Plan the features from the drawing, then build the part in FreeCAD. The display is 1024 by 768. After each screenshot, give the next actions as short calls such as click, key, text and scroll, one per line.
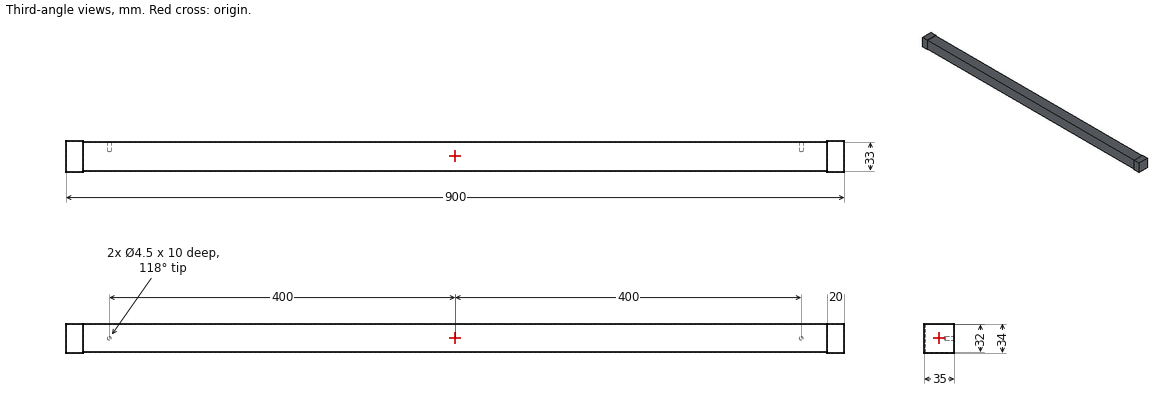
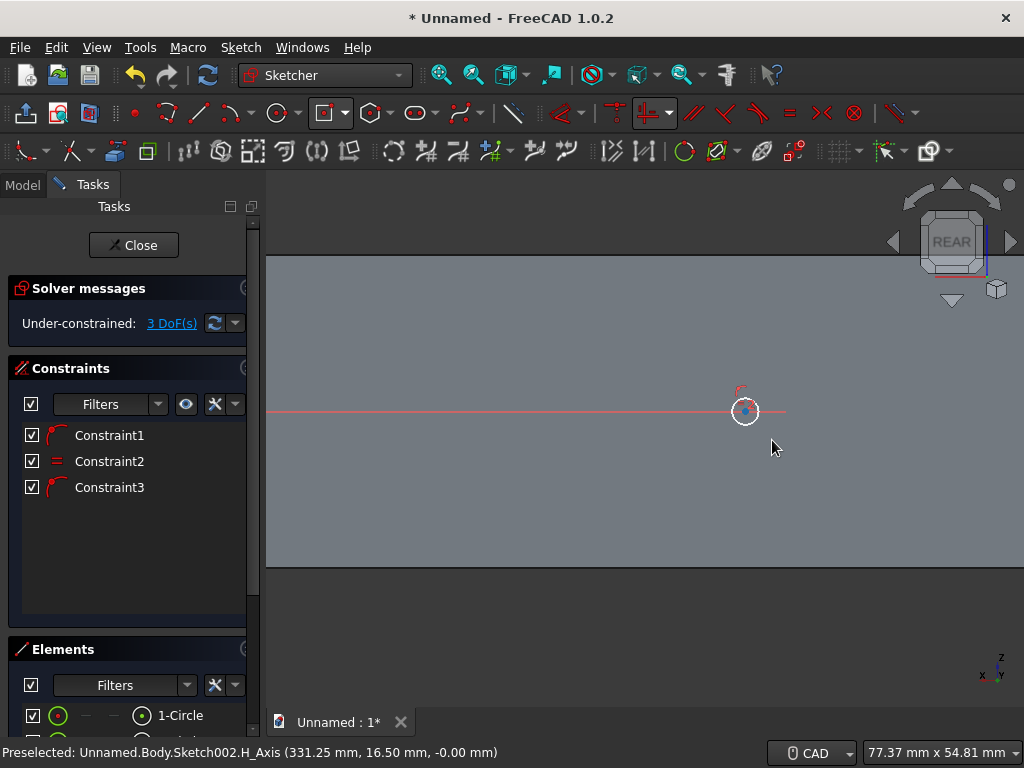
click(755, 421)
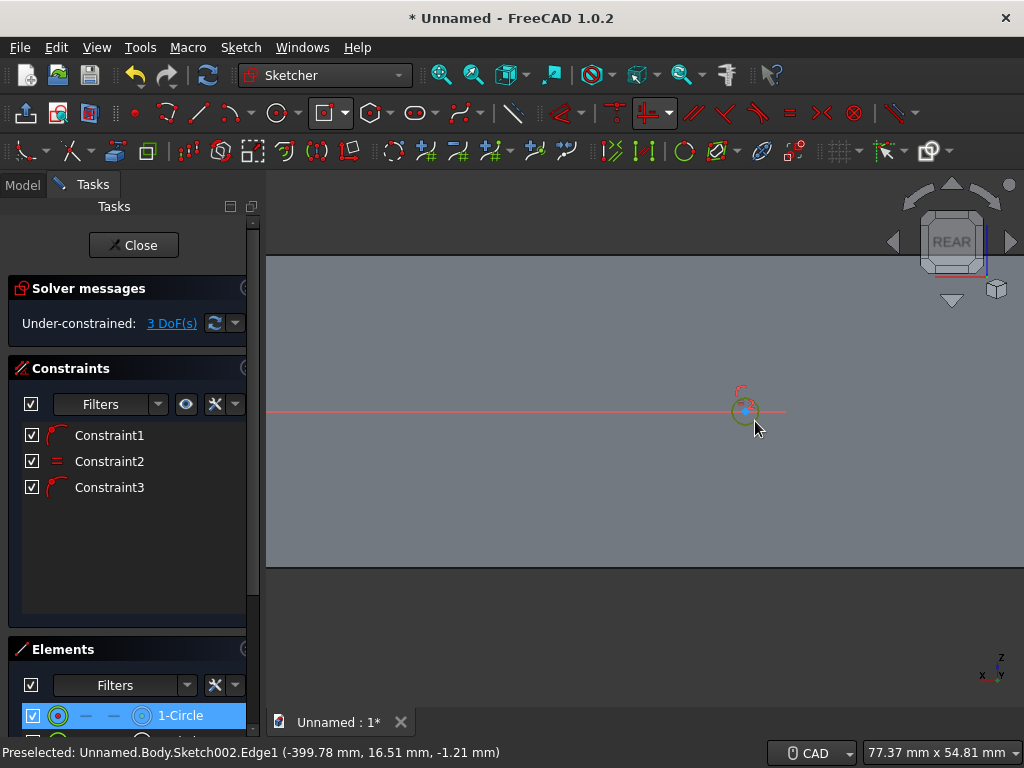
key(k)
key(o)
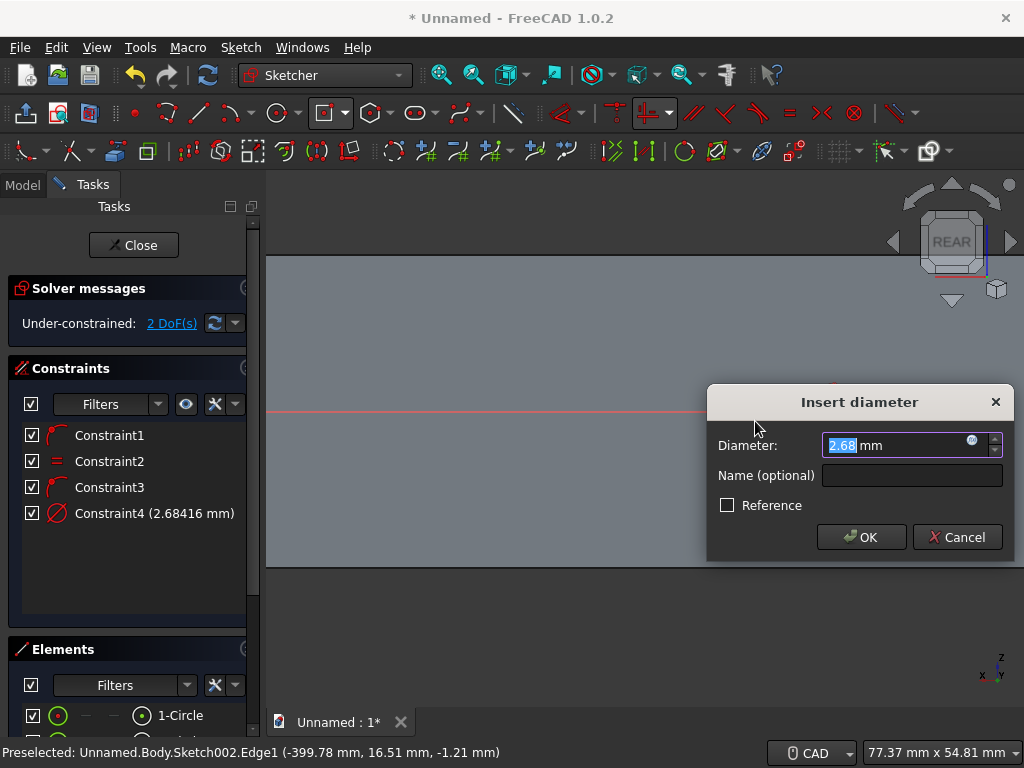
text(4.5)
key(Return)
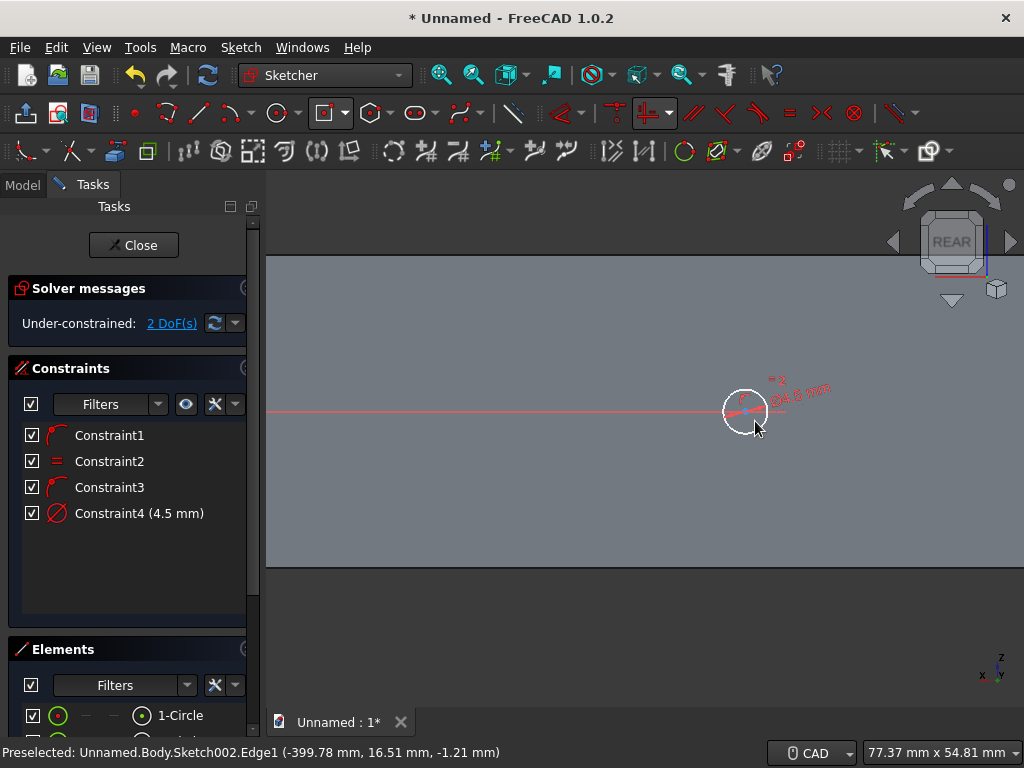
scroll(773, 440, down, 15)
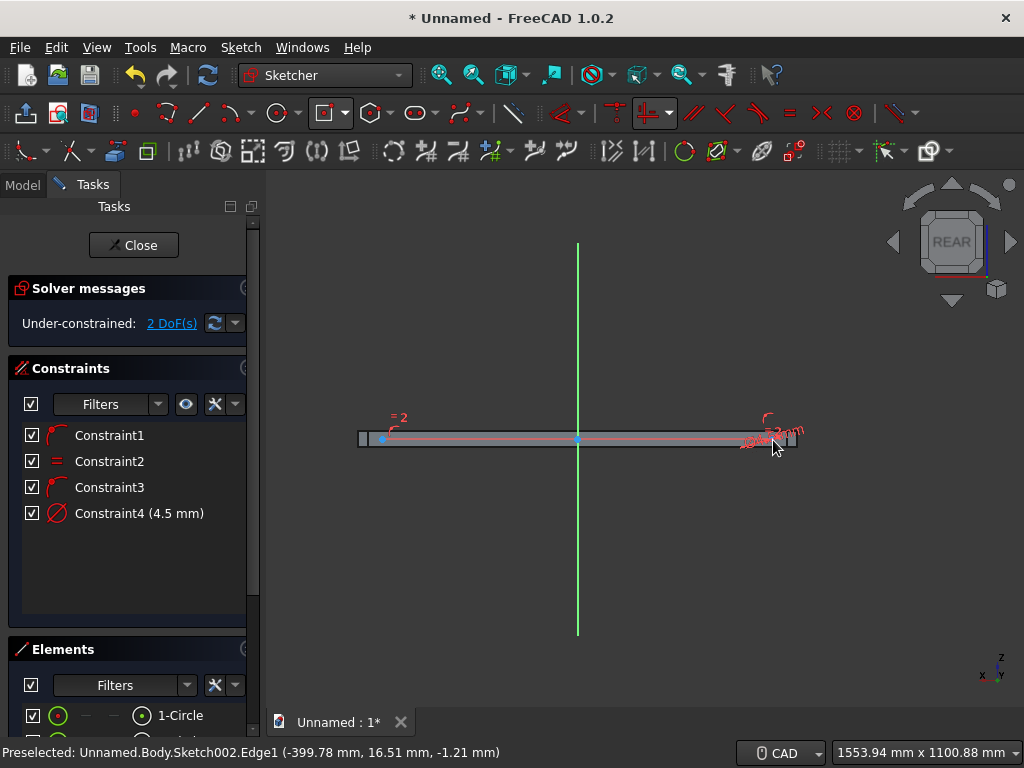
click(772, 439)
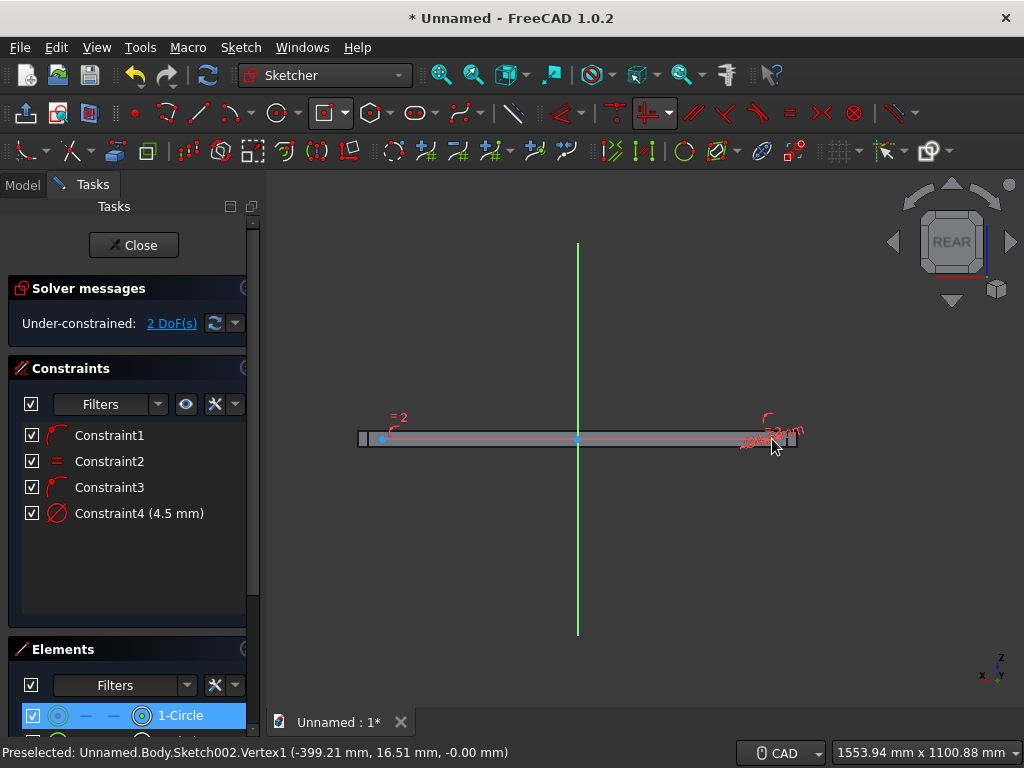
key(l)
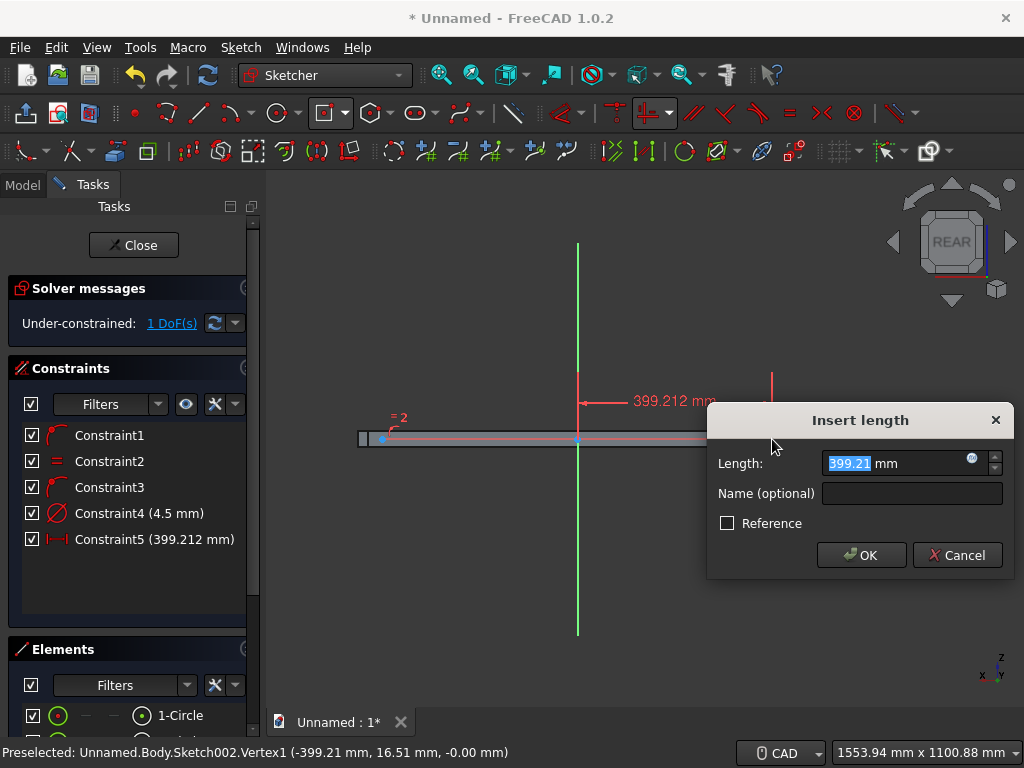
text(400)
key(Return)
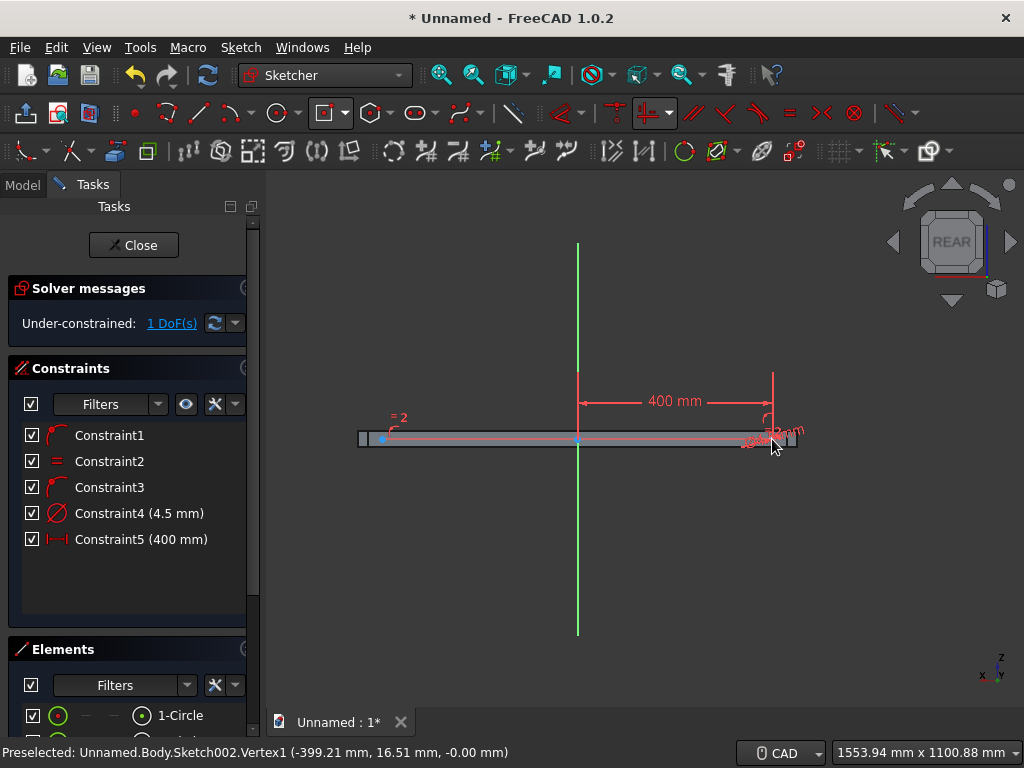
click(382, 439)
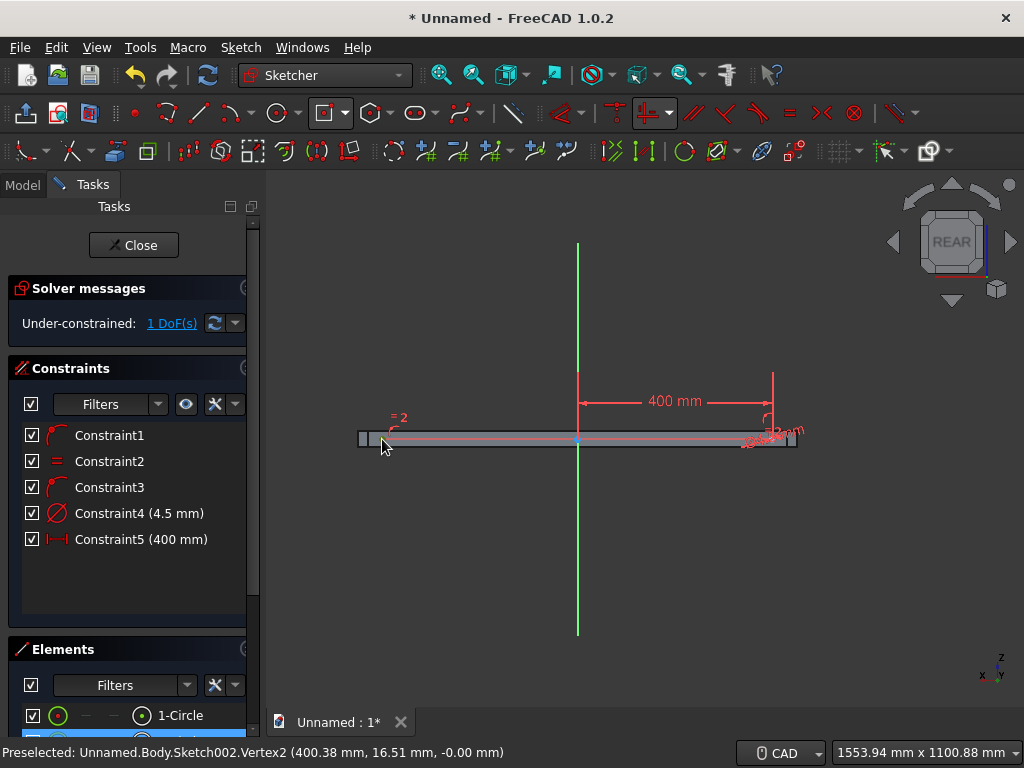
key(l)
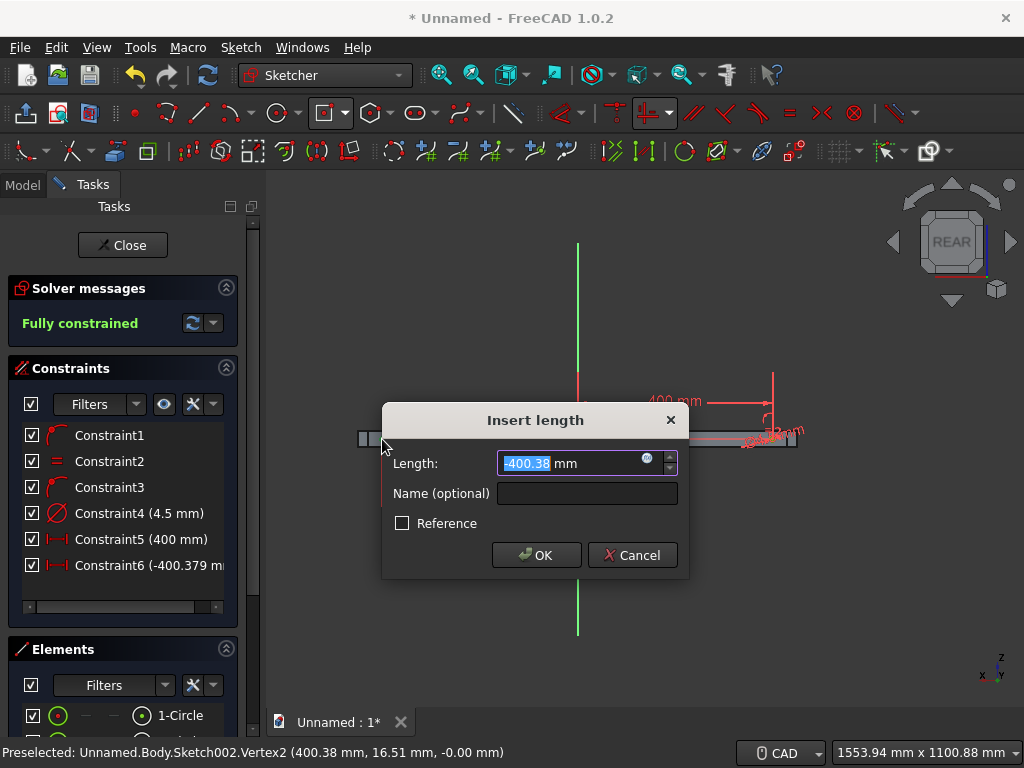
text(-400)
key(Return)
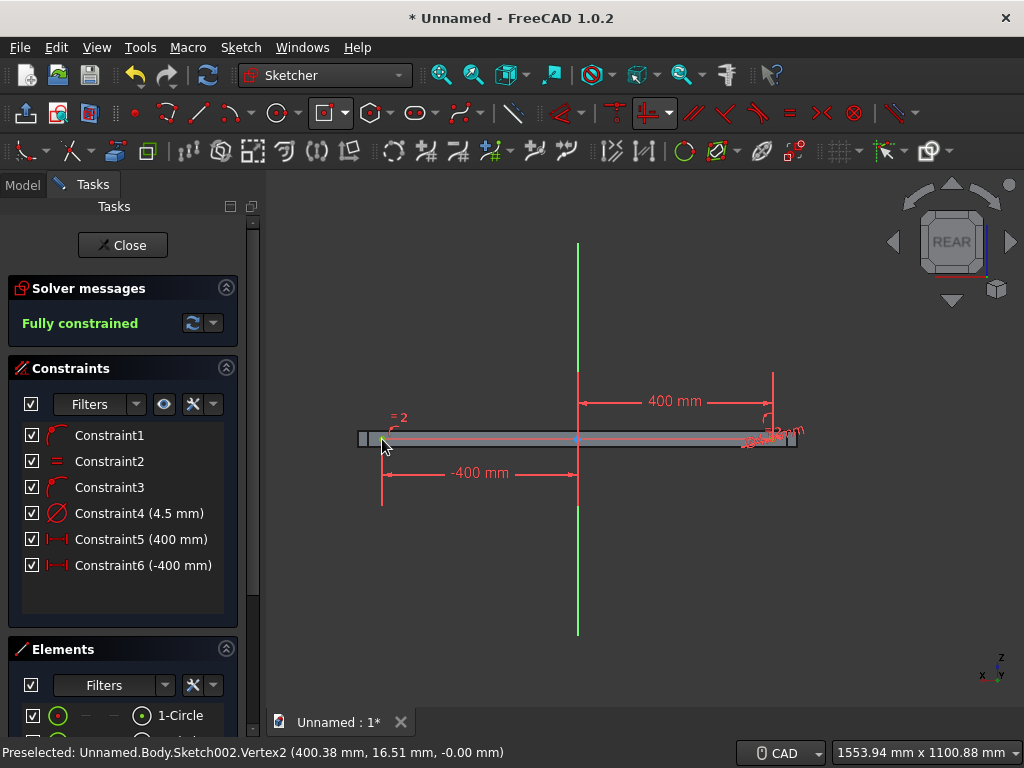
click(123, 245)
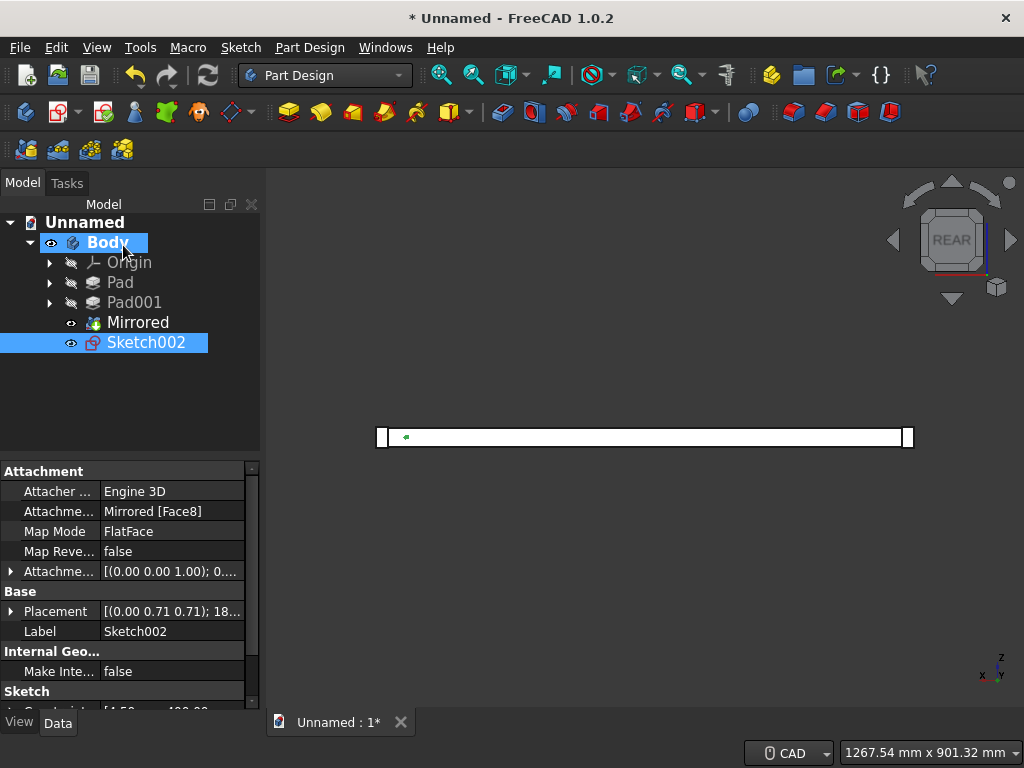
click(536, 112)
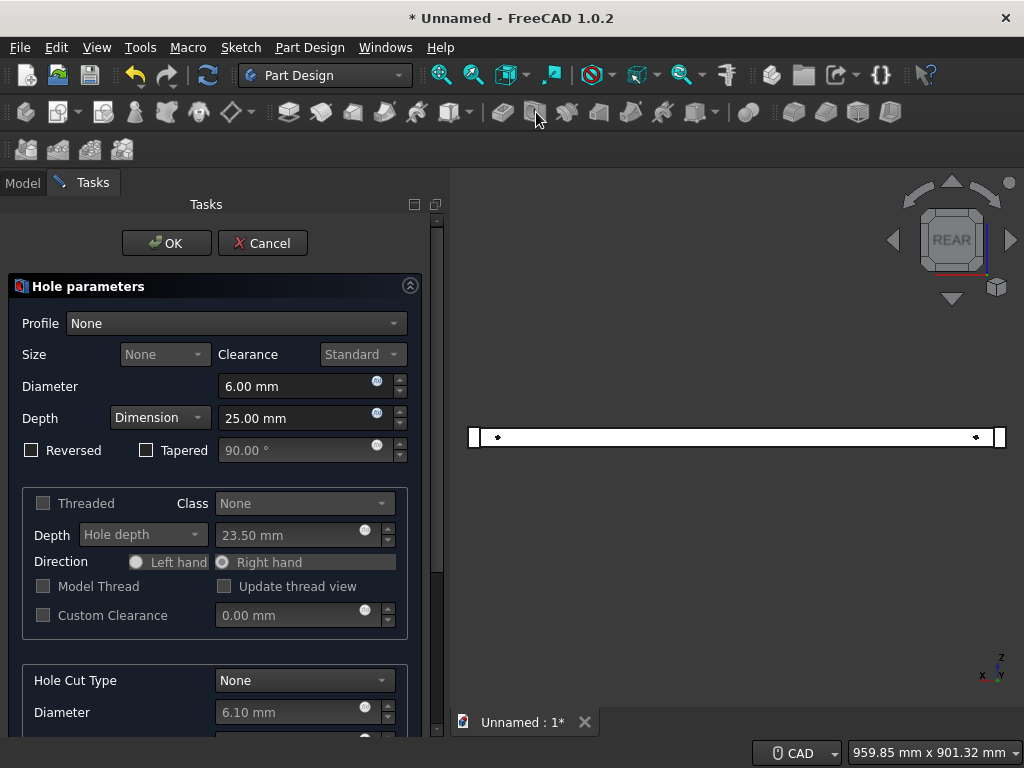
triple_click(305, 386)